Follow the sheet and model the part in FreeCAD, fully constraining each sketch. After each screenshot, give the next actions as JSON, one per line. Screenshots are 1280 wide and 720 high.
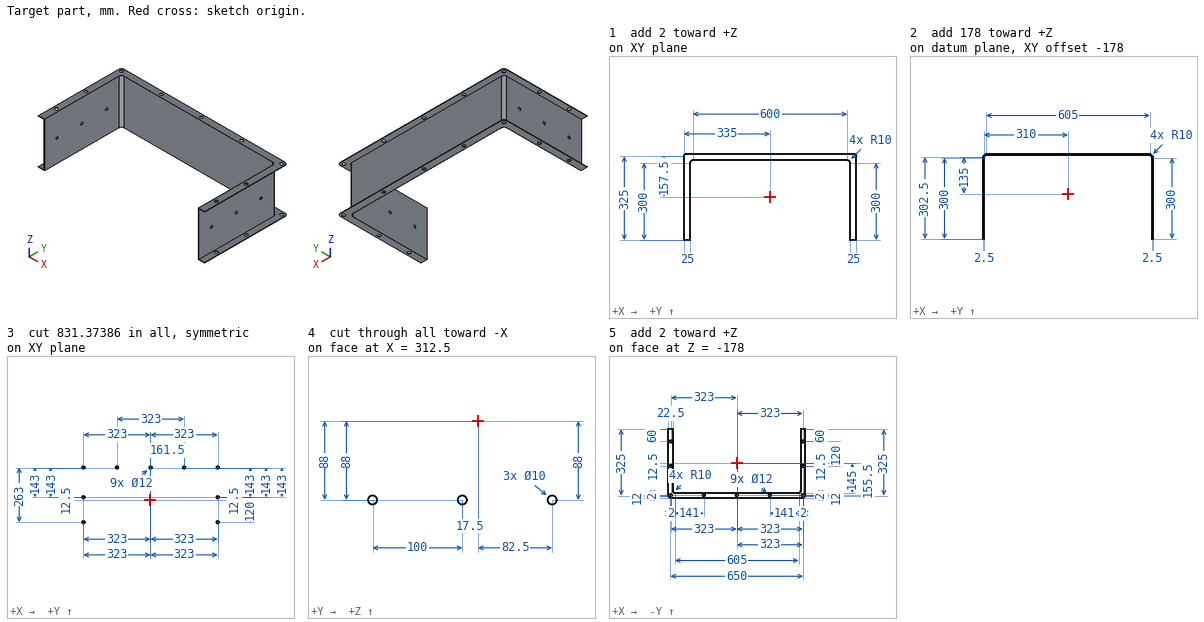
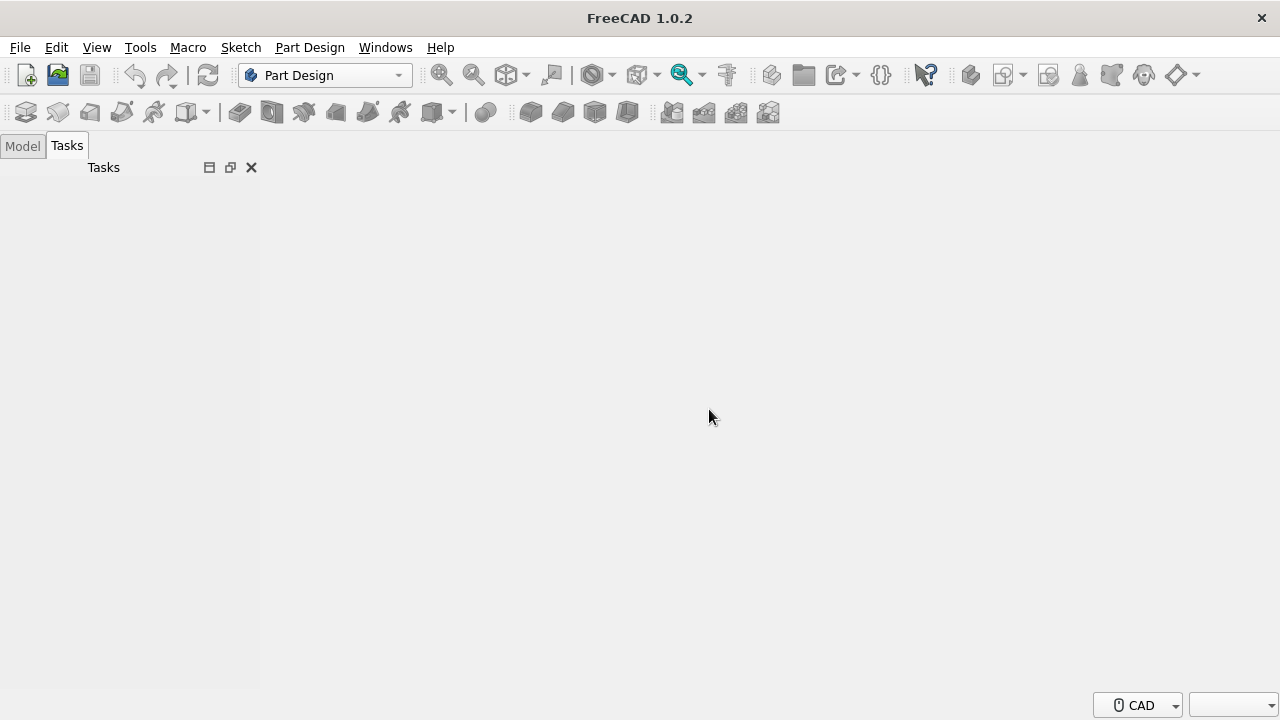
{"action": "left_click", "coordinate": [26, 76]}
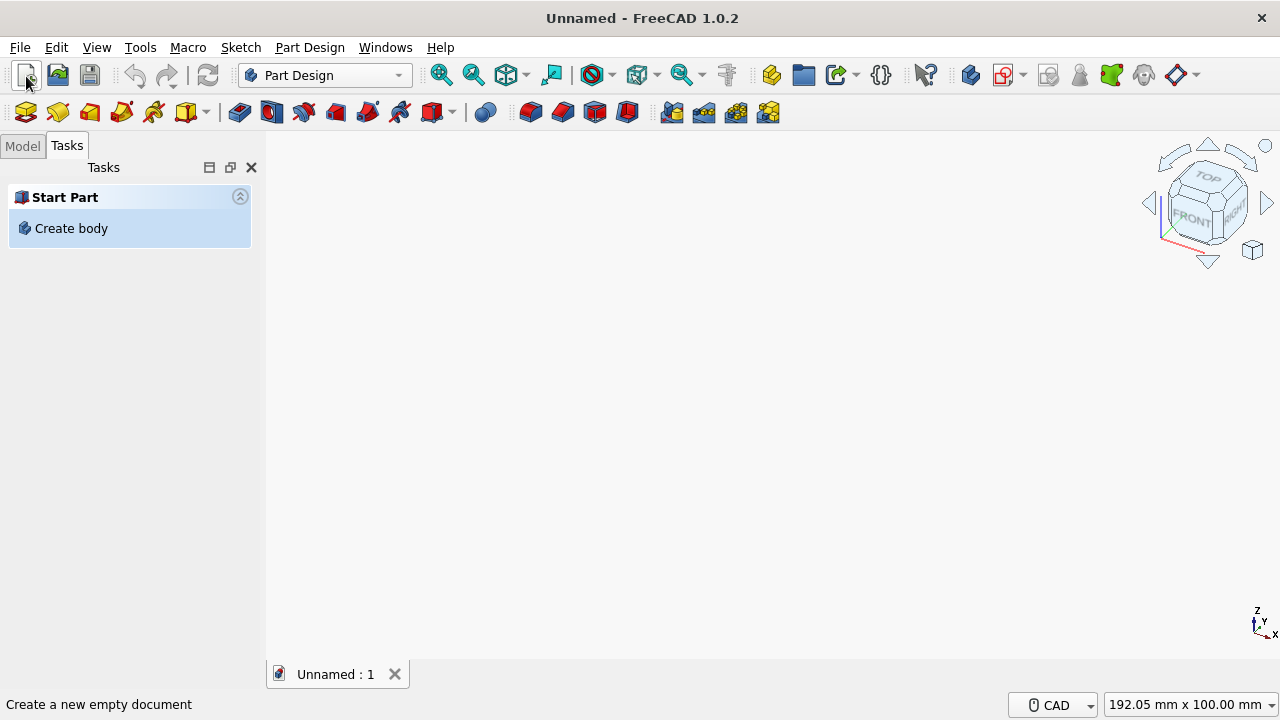
{"action": "left_click", "coordinate": [1004, 76]}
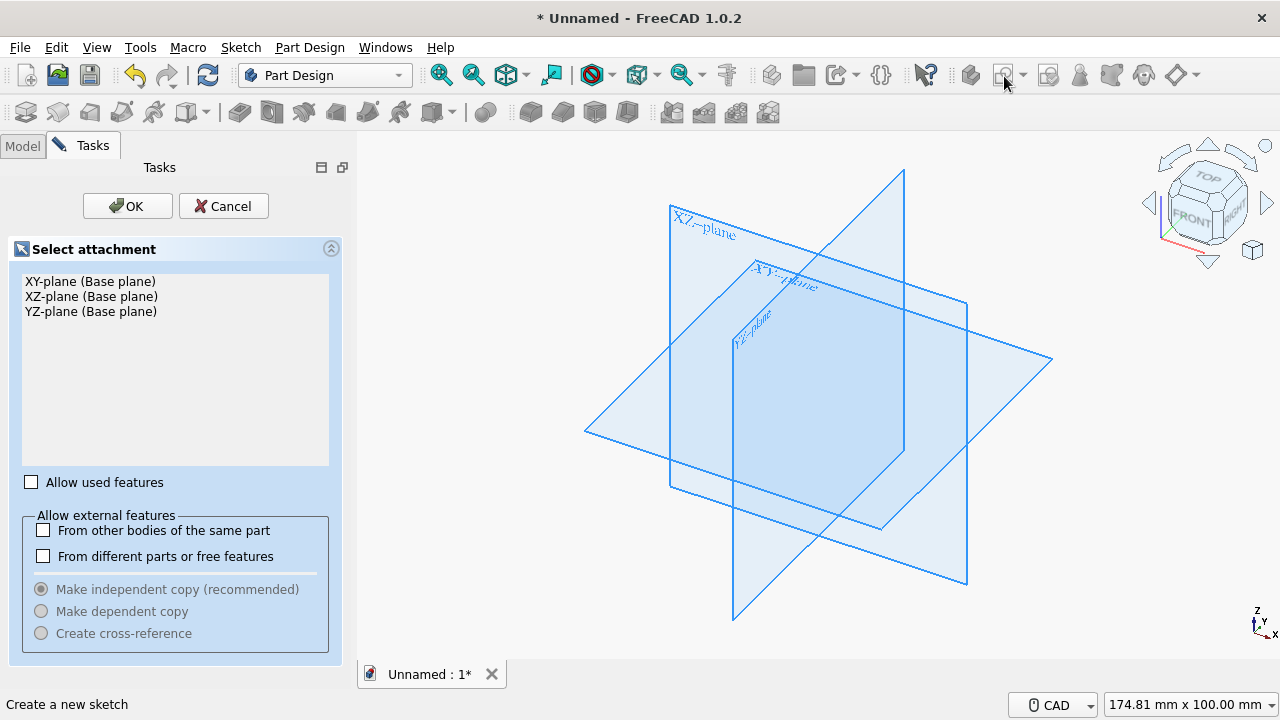
{"action": "left_click", "coordinate": [82, 282]}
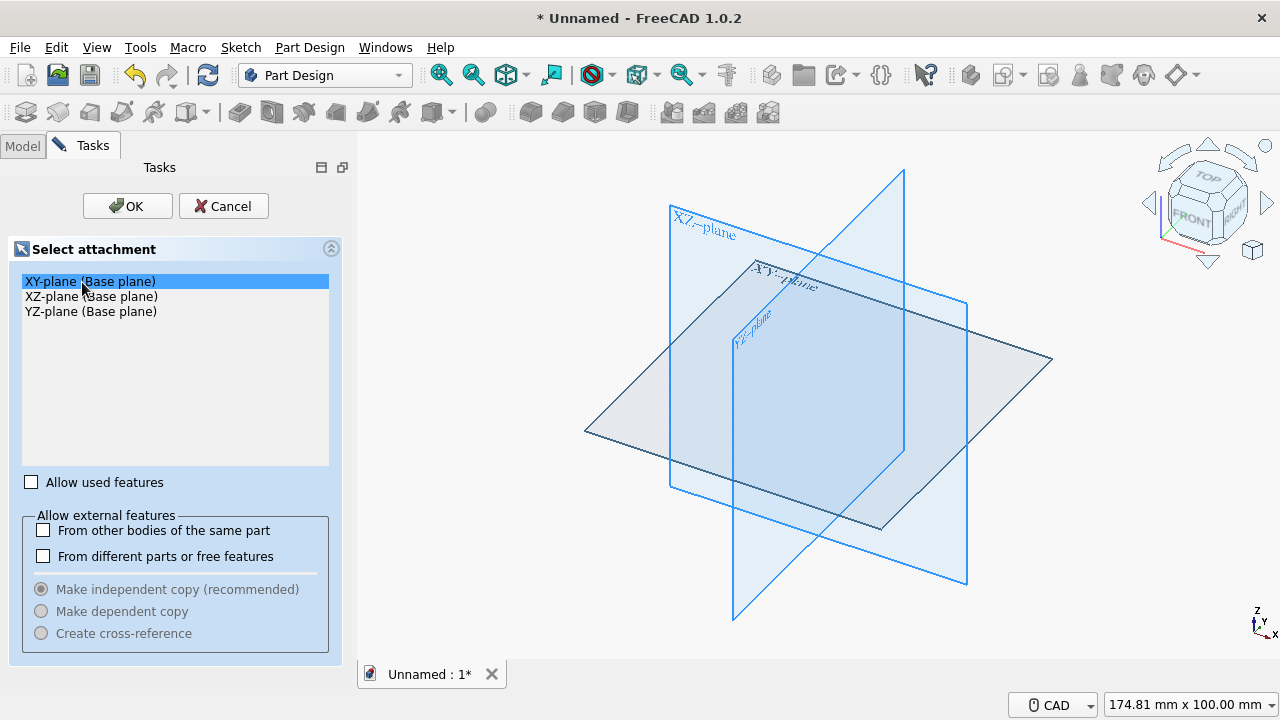
{"action": "left_click", "coordinate": [128, 206]}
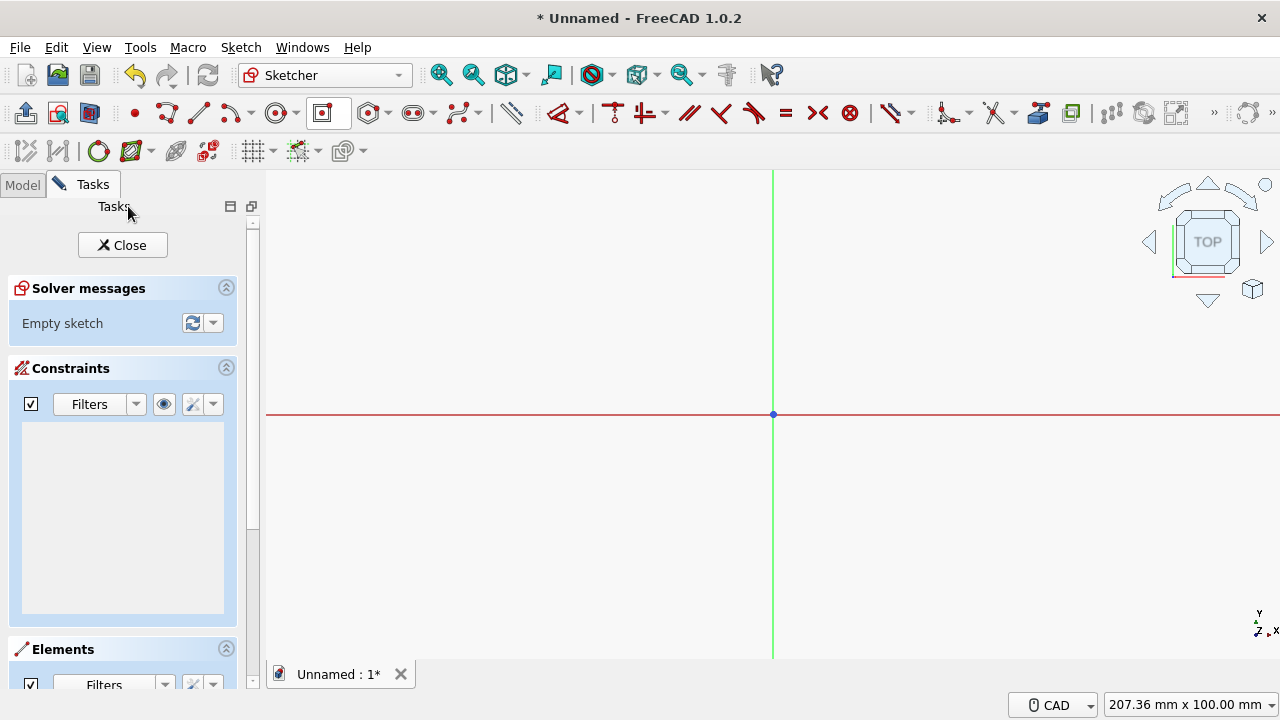
{"action": "scroll", "coordinate": [691, 415], "scroll_direction": "down", "scroll_amount": 9}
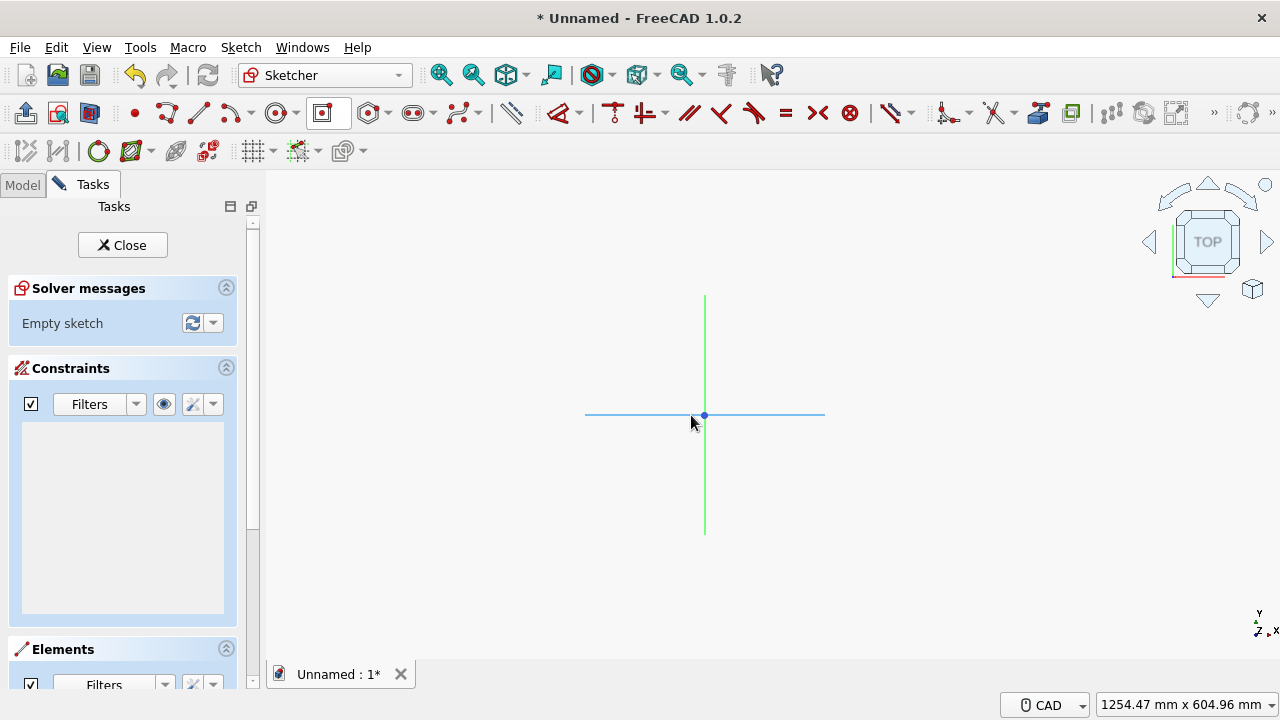
{"action": "left_click", "coordinate": [168, 114]}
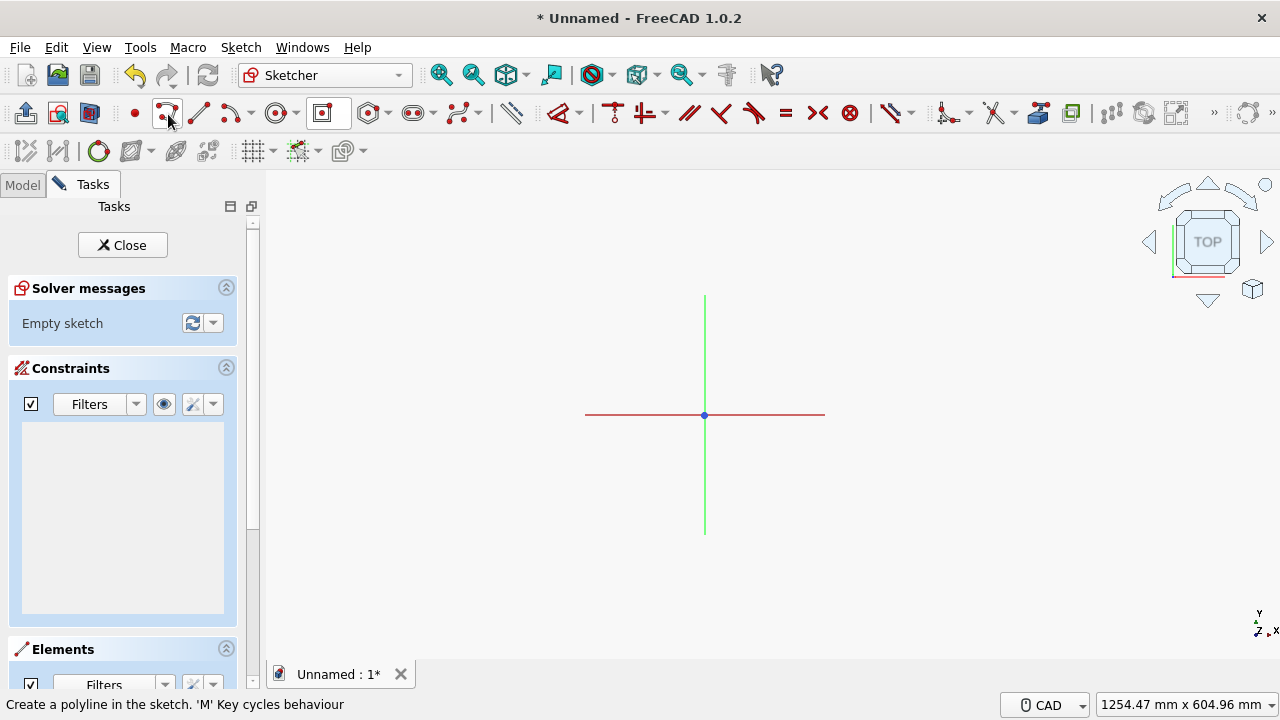
{"action": "left_click", "coordinate": [434, 288]}
{"action": "left_click", "coordinate": [434, 551]}
{"action": "left_click", "coordinate": [454, 551]}
{"action": "left_click", "coordinate": [454, 308]}
{"action": "right_click", "coordinate": [454, 308]}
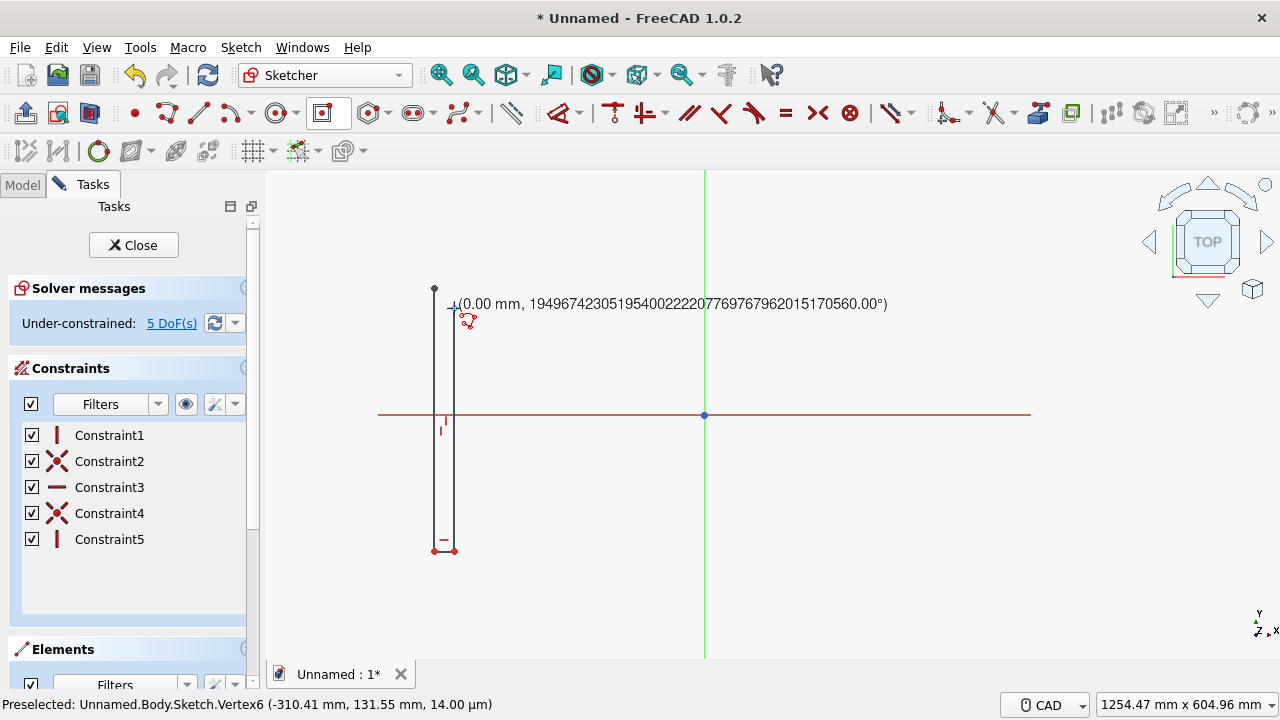
{"action": "left_click", "coordinate": [200, 114]}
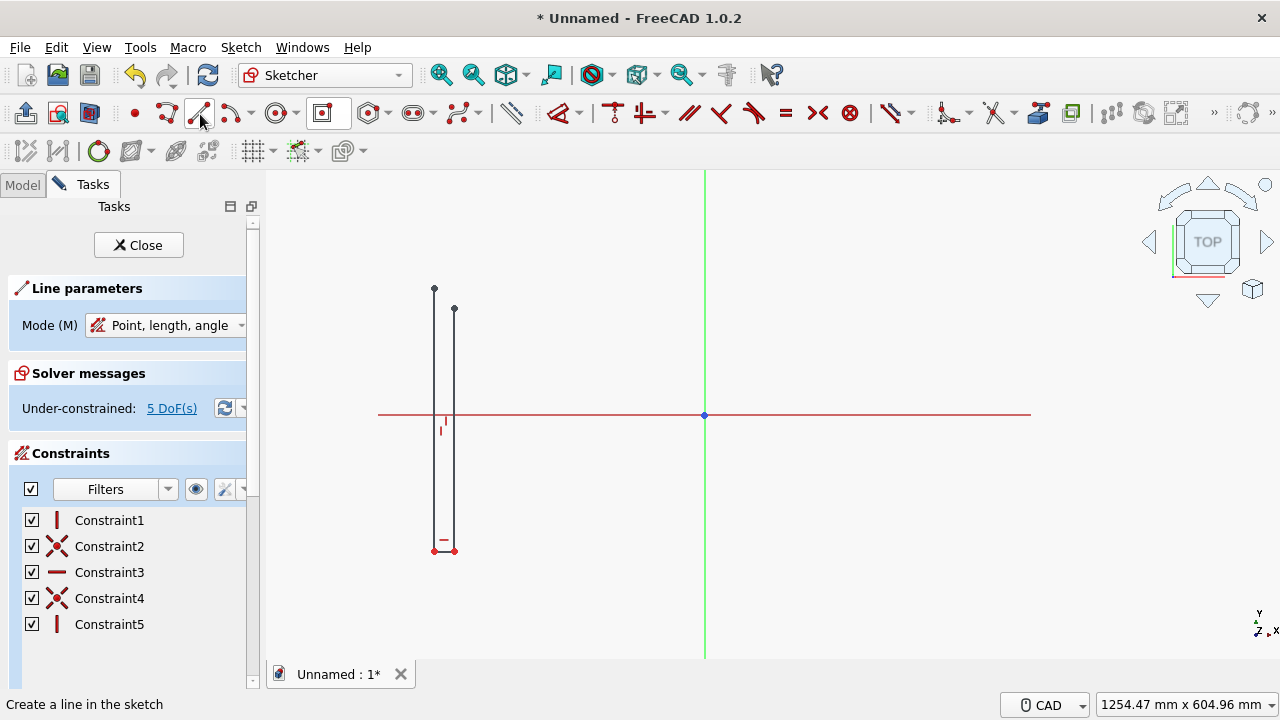
{"action": "scroll", "coordinate": [462, 300], "scroll_direction": "up", "scroll_amount": 2}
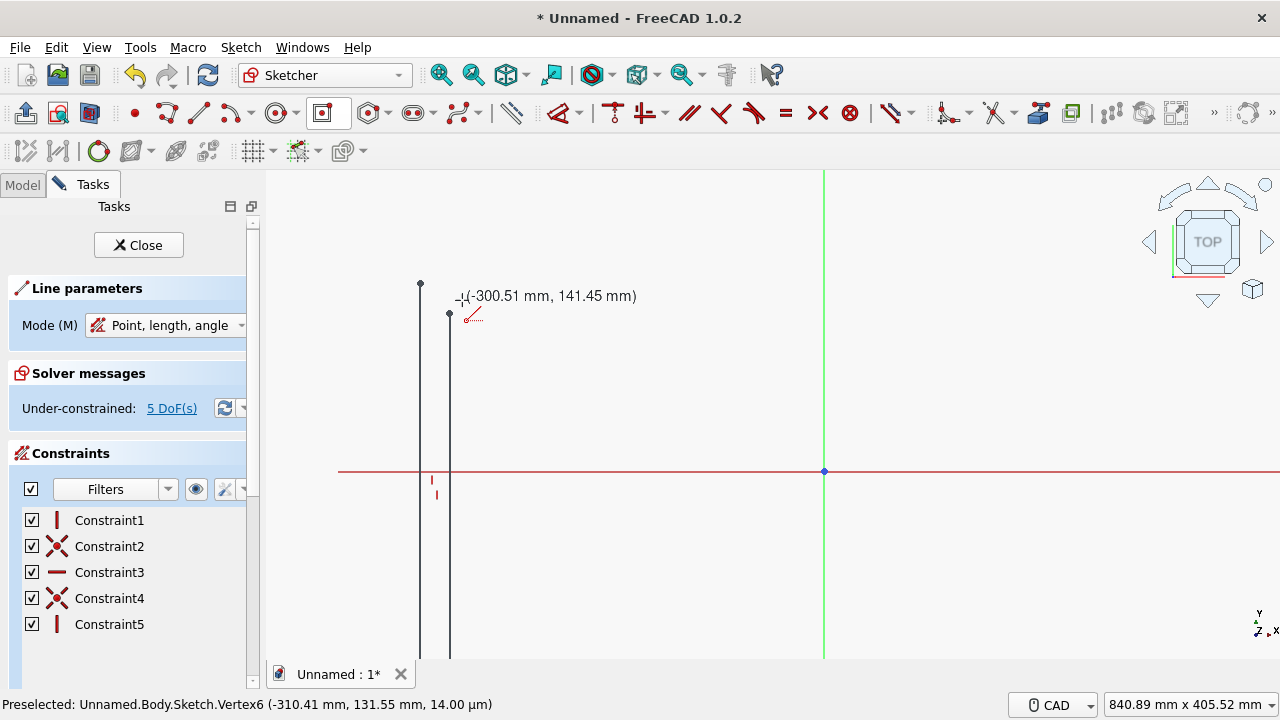
{"action": "left_click", "coordinate": [463, 300]}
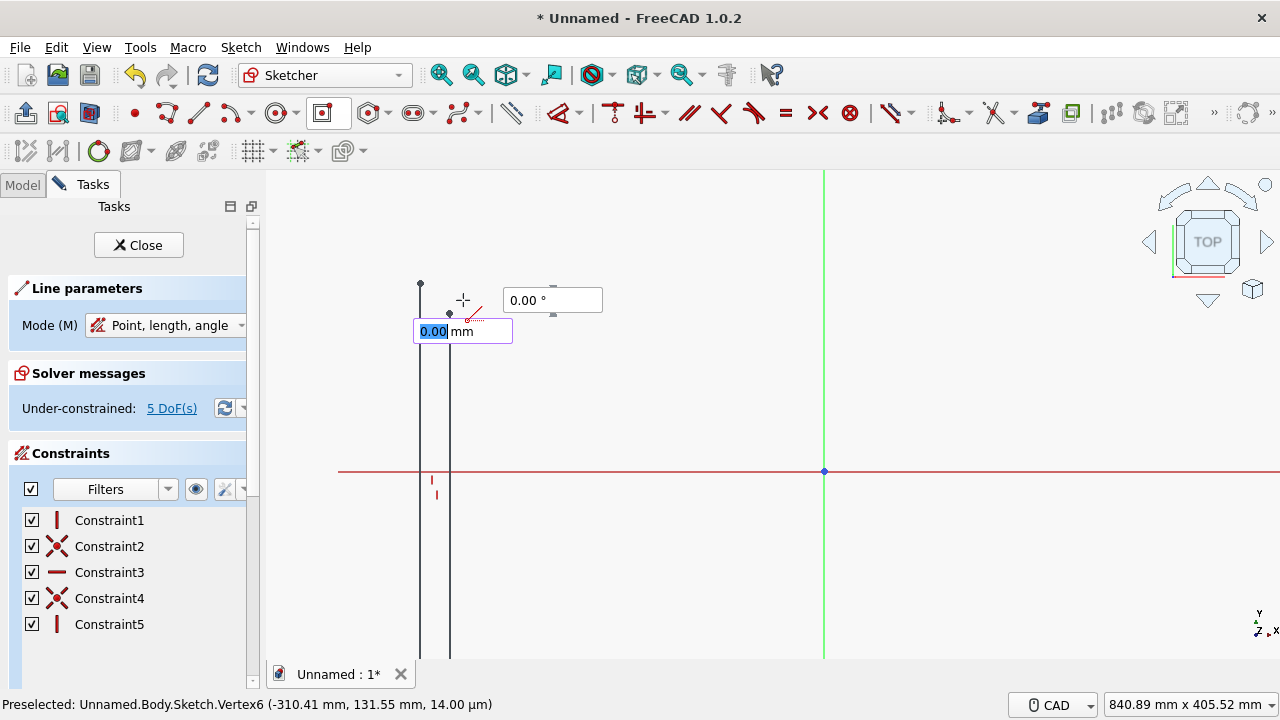
{"action": "scroll", "coordinate": [461, 298], "scroll_direction": "down", "scroll_amount": 2}